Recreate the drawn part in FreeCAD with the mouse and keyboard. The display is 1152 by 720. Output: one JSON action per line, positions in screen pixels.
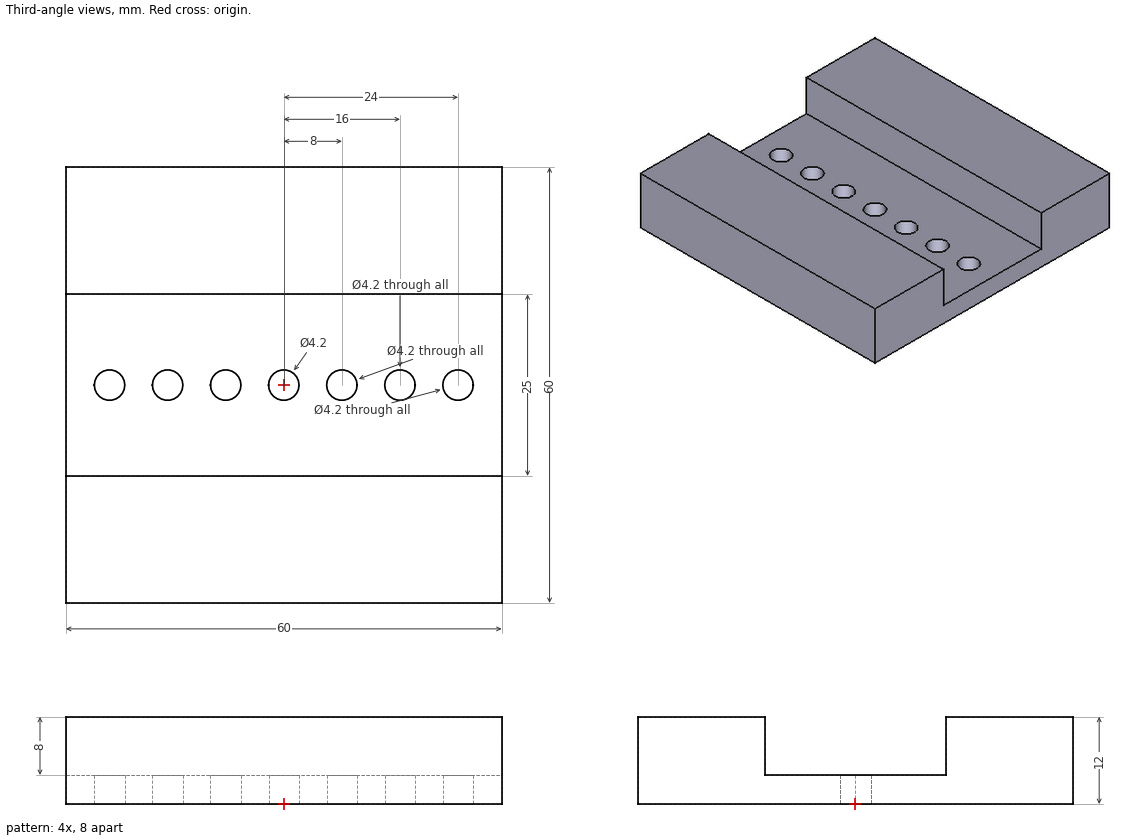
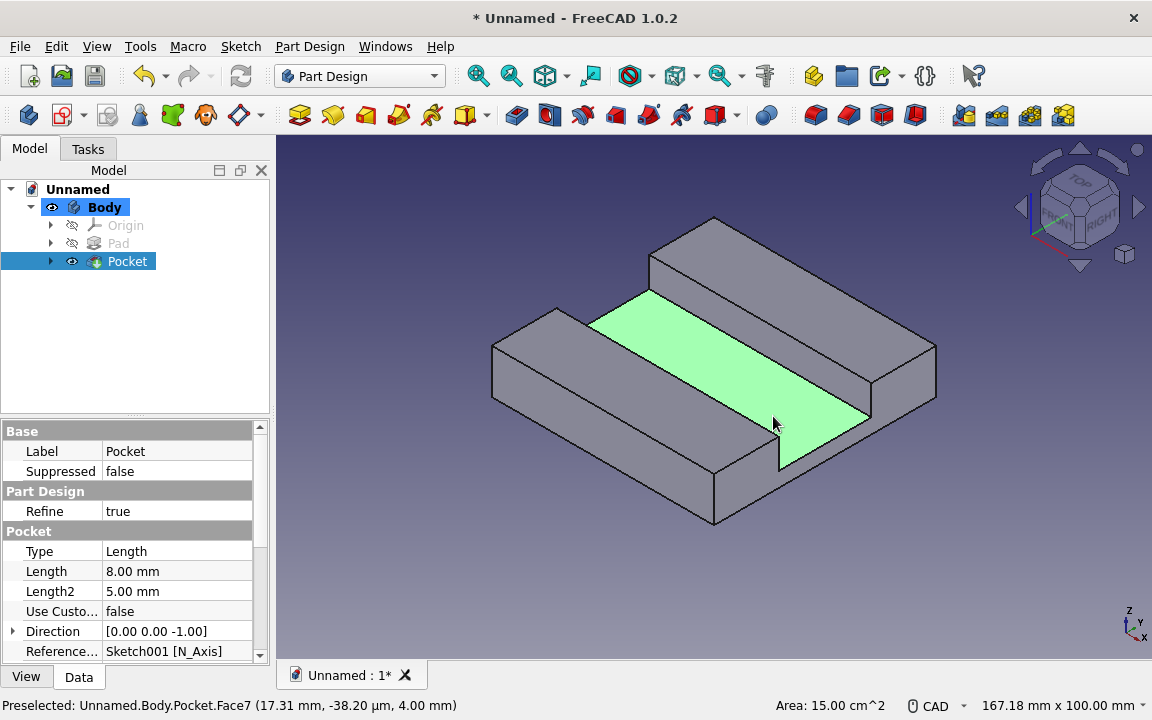
{"action": "left_click", "coordinate": [62, 116]}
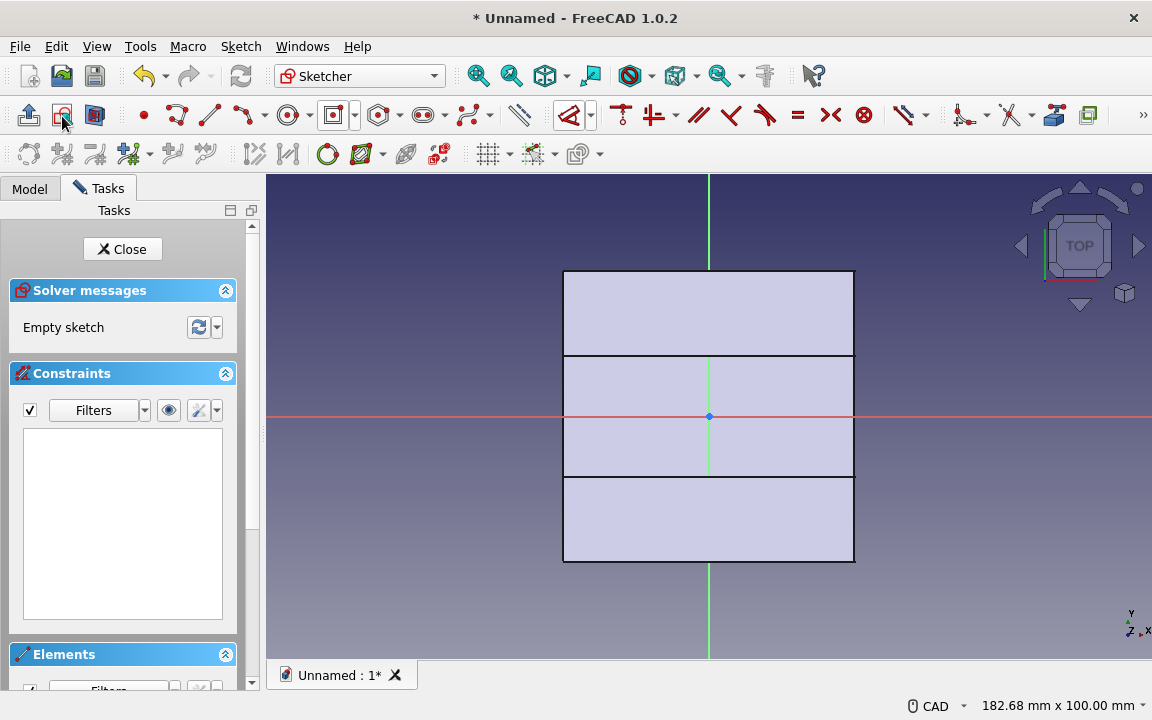
{"action": "scroll", "coordinate": [714, 416], "scroll_direction": "up", "scroll_amount": 13}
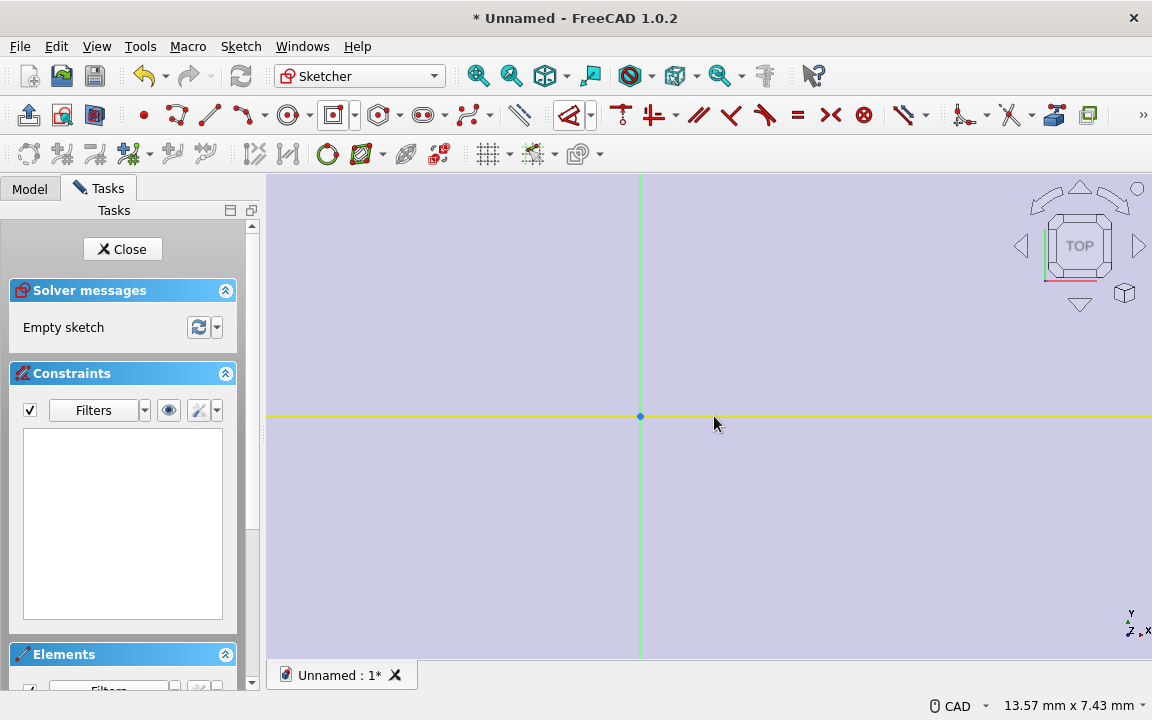
{"action": "left_click", "coordinate": [288, 116]}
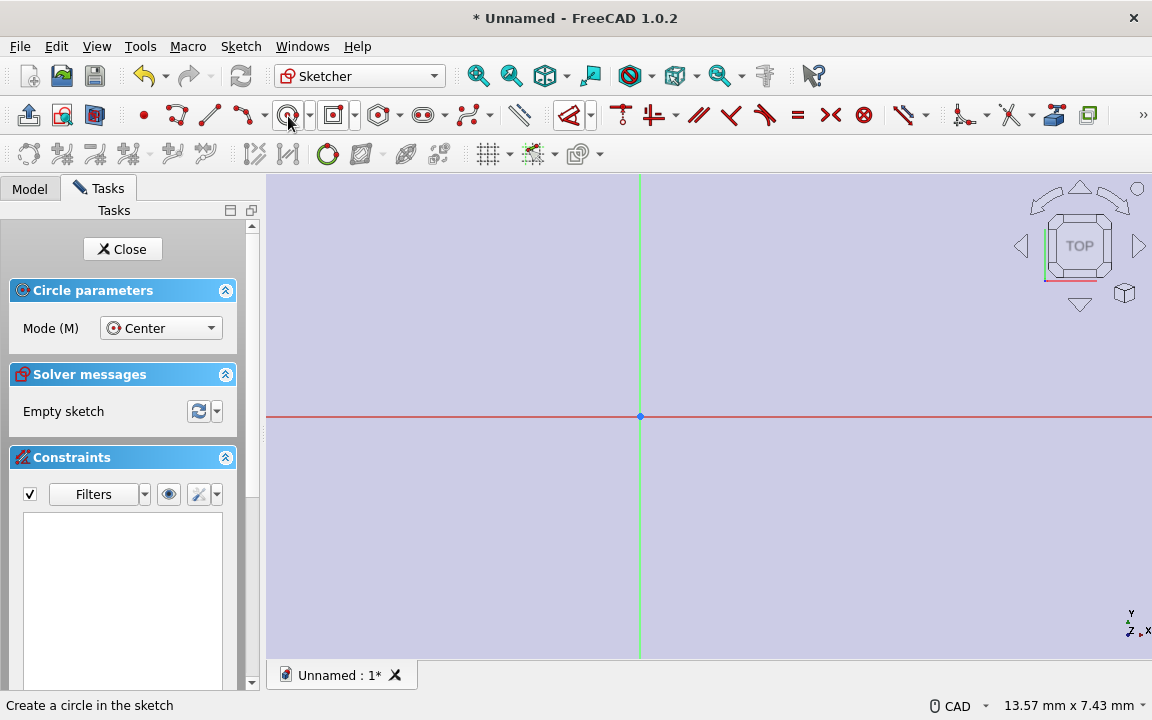
{"action": "left_click", "coordinate": [640, 416]}
{"action": "mouse_move", "coordinate": [737, 320]}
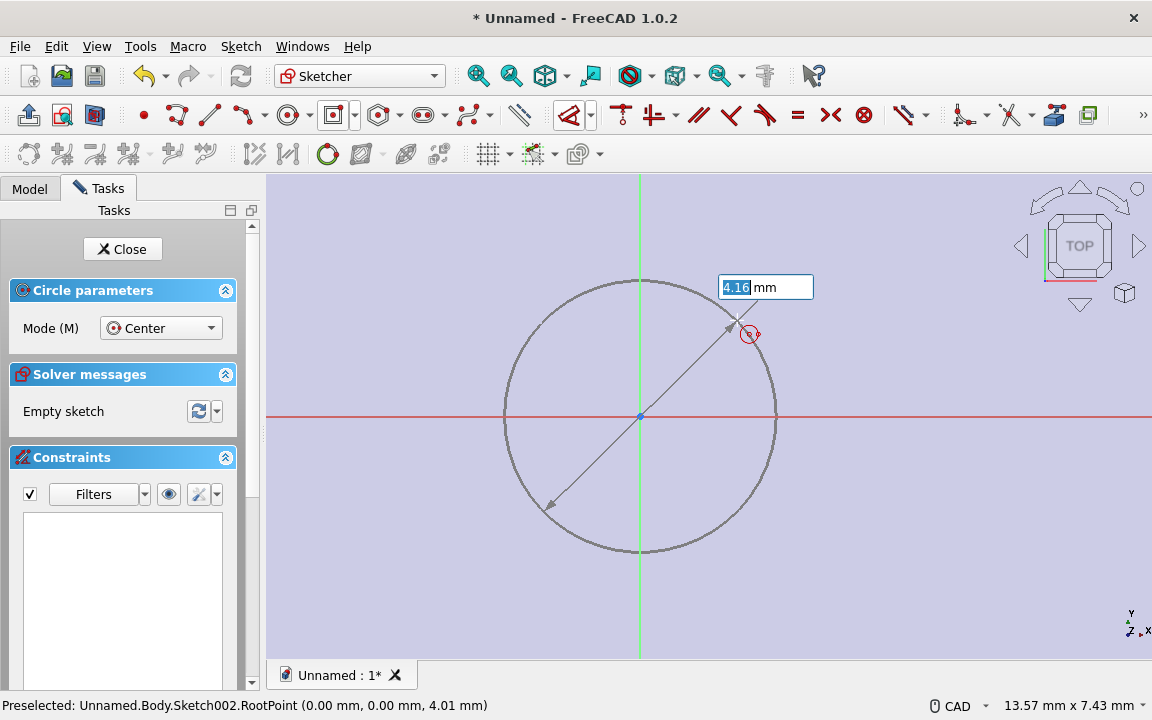
{"action": "type", "text": "4.2"}
{"action": "key", "text": "Return"}
{"action": "key", "text": "Escape"}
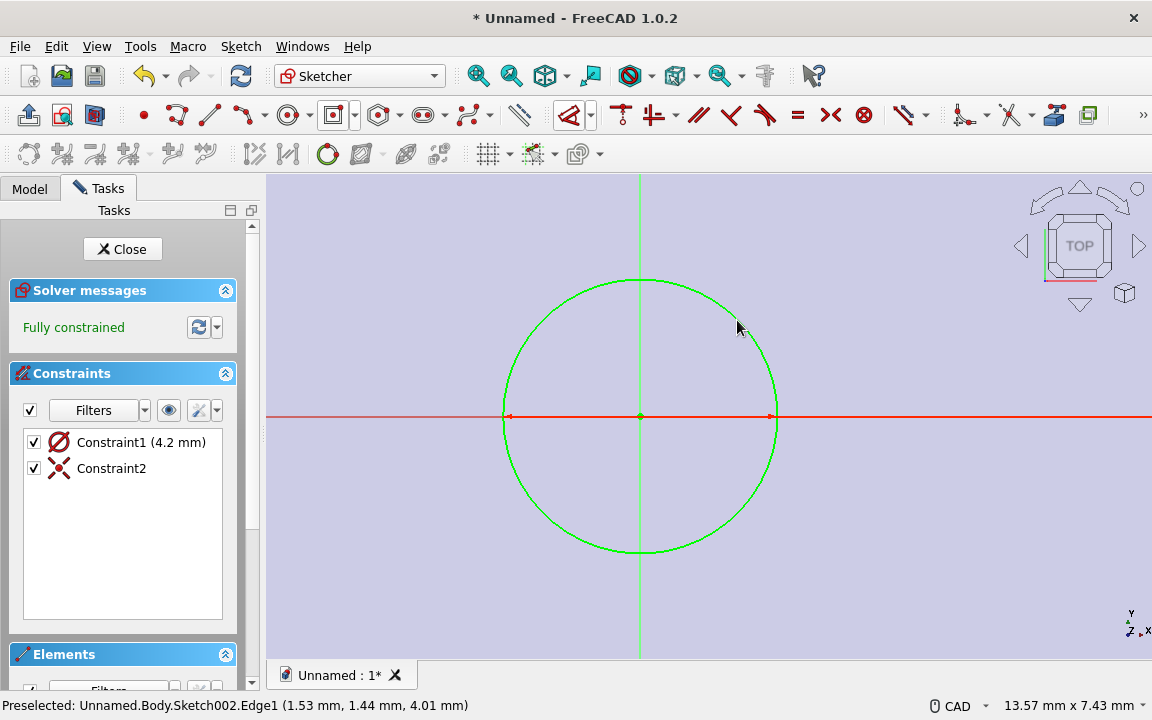
{"action": "left_click", "coordinate": [123, 249]}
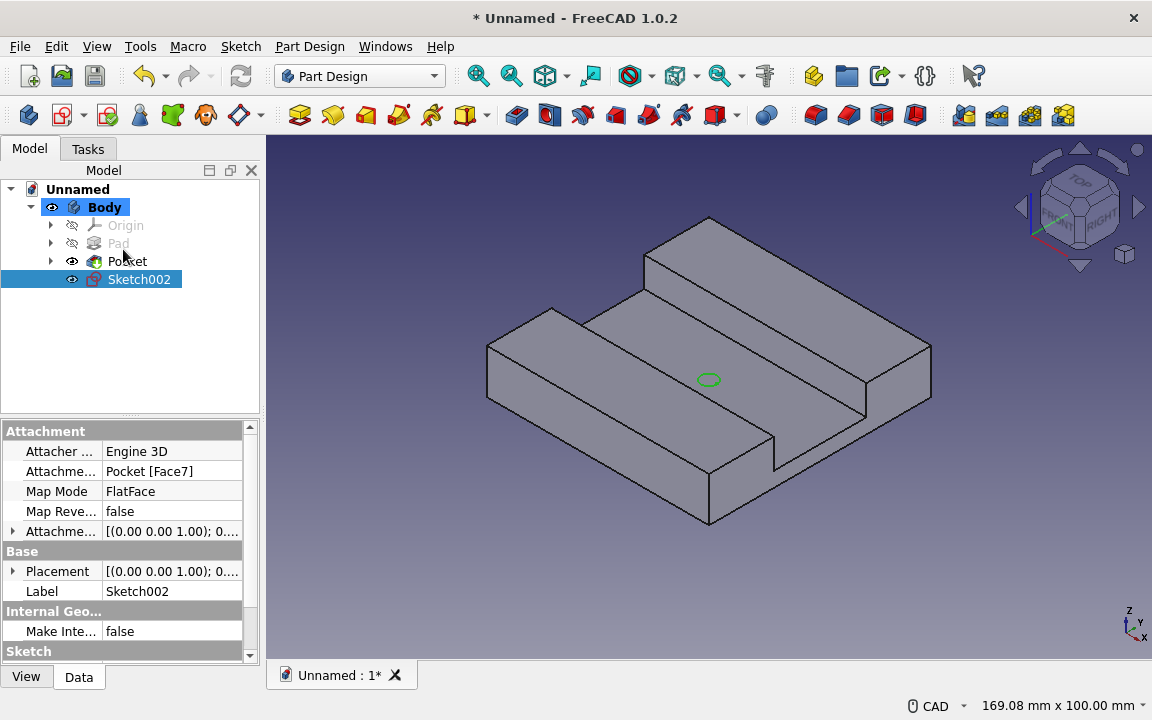
{"action": "left_click", "coordinate": [517, 116]}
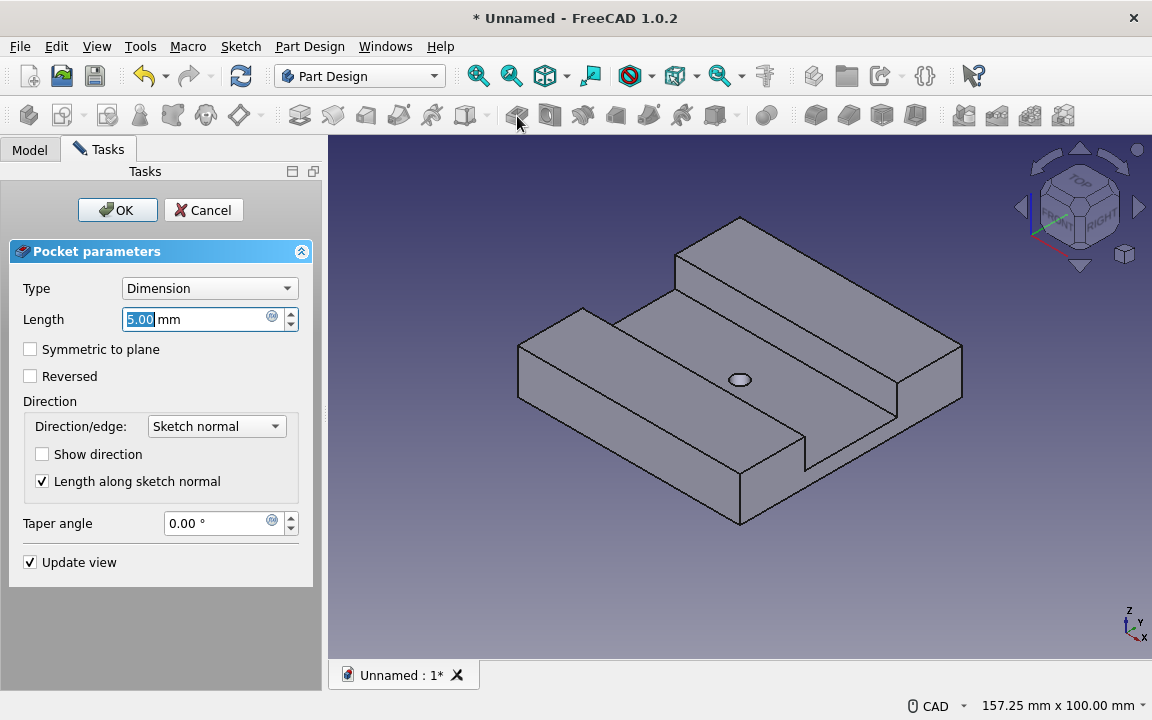
{"action": "left_click", "coordinate": [210, 288]}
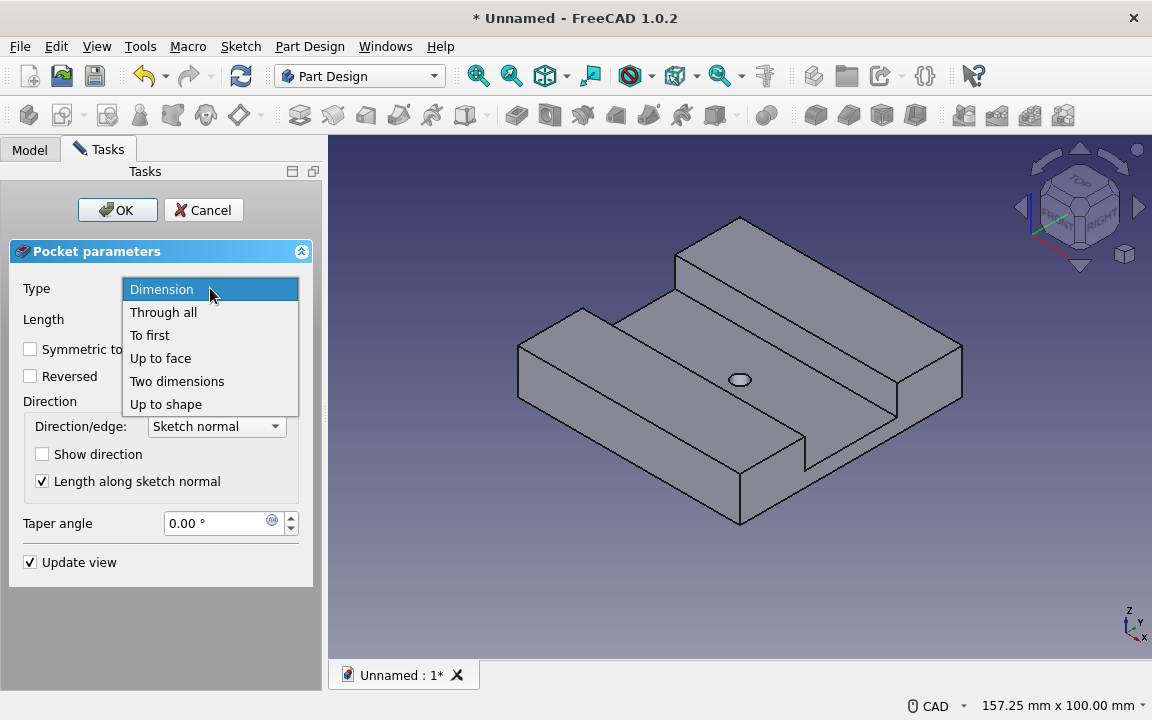
{"action": "left_click", "coordinate": [208, 312]}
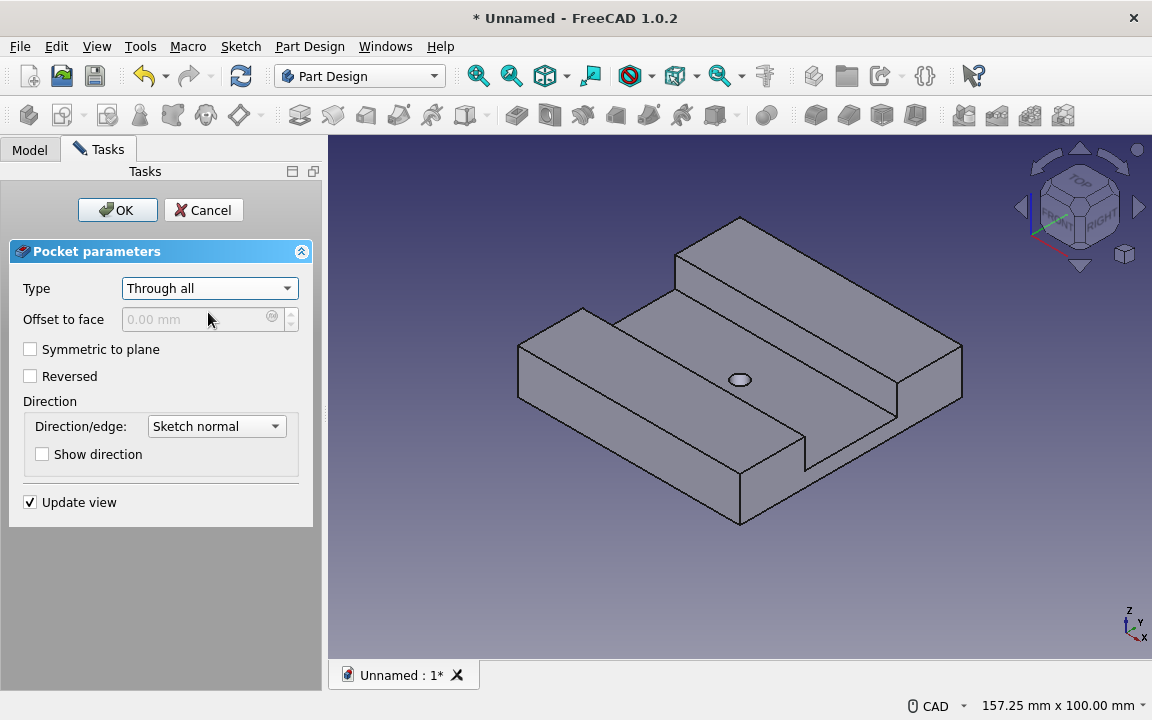
{"action": "left_click", "coordinate": [118, 210]}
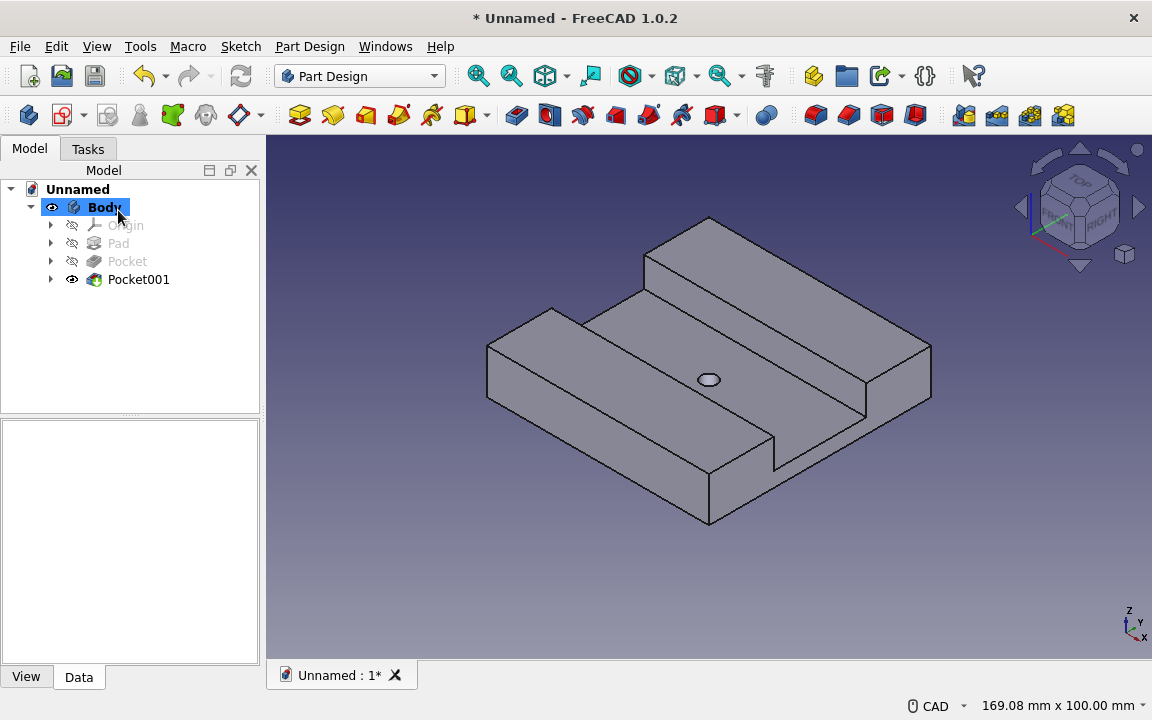
{"action": "left_click", "coordinate": [117, 279]}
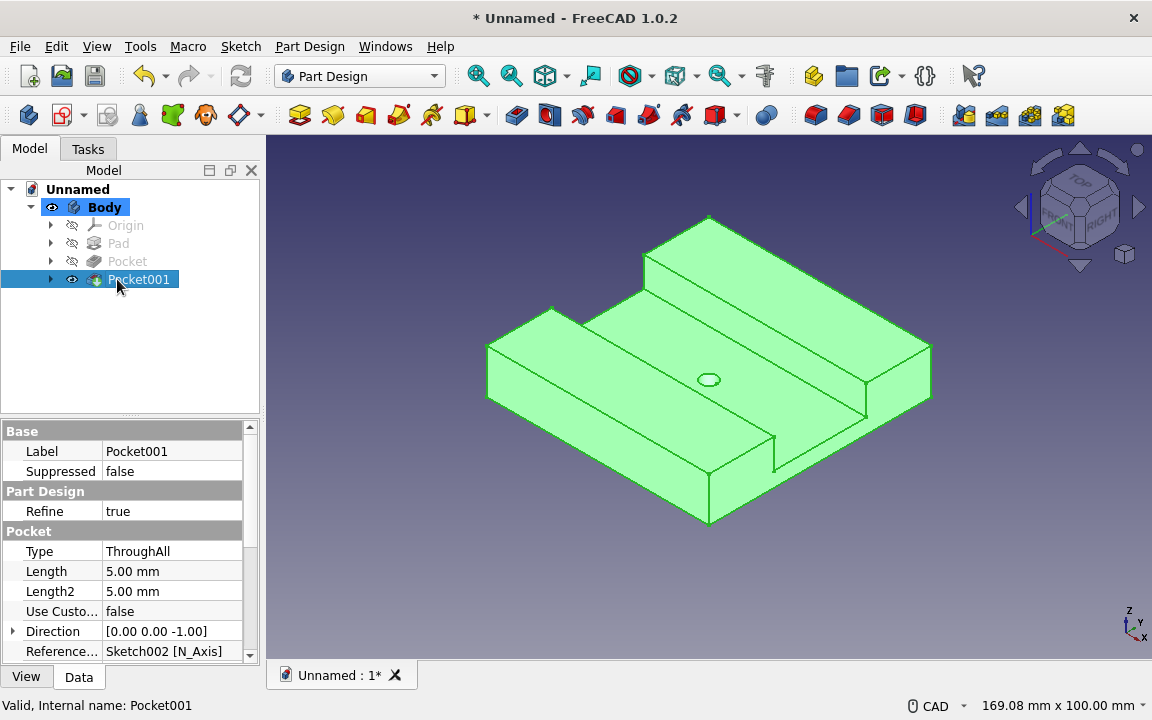
{"action": "left_click", "coordinate": [997, 116]}